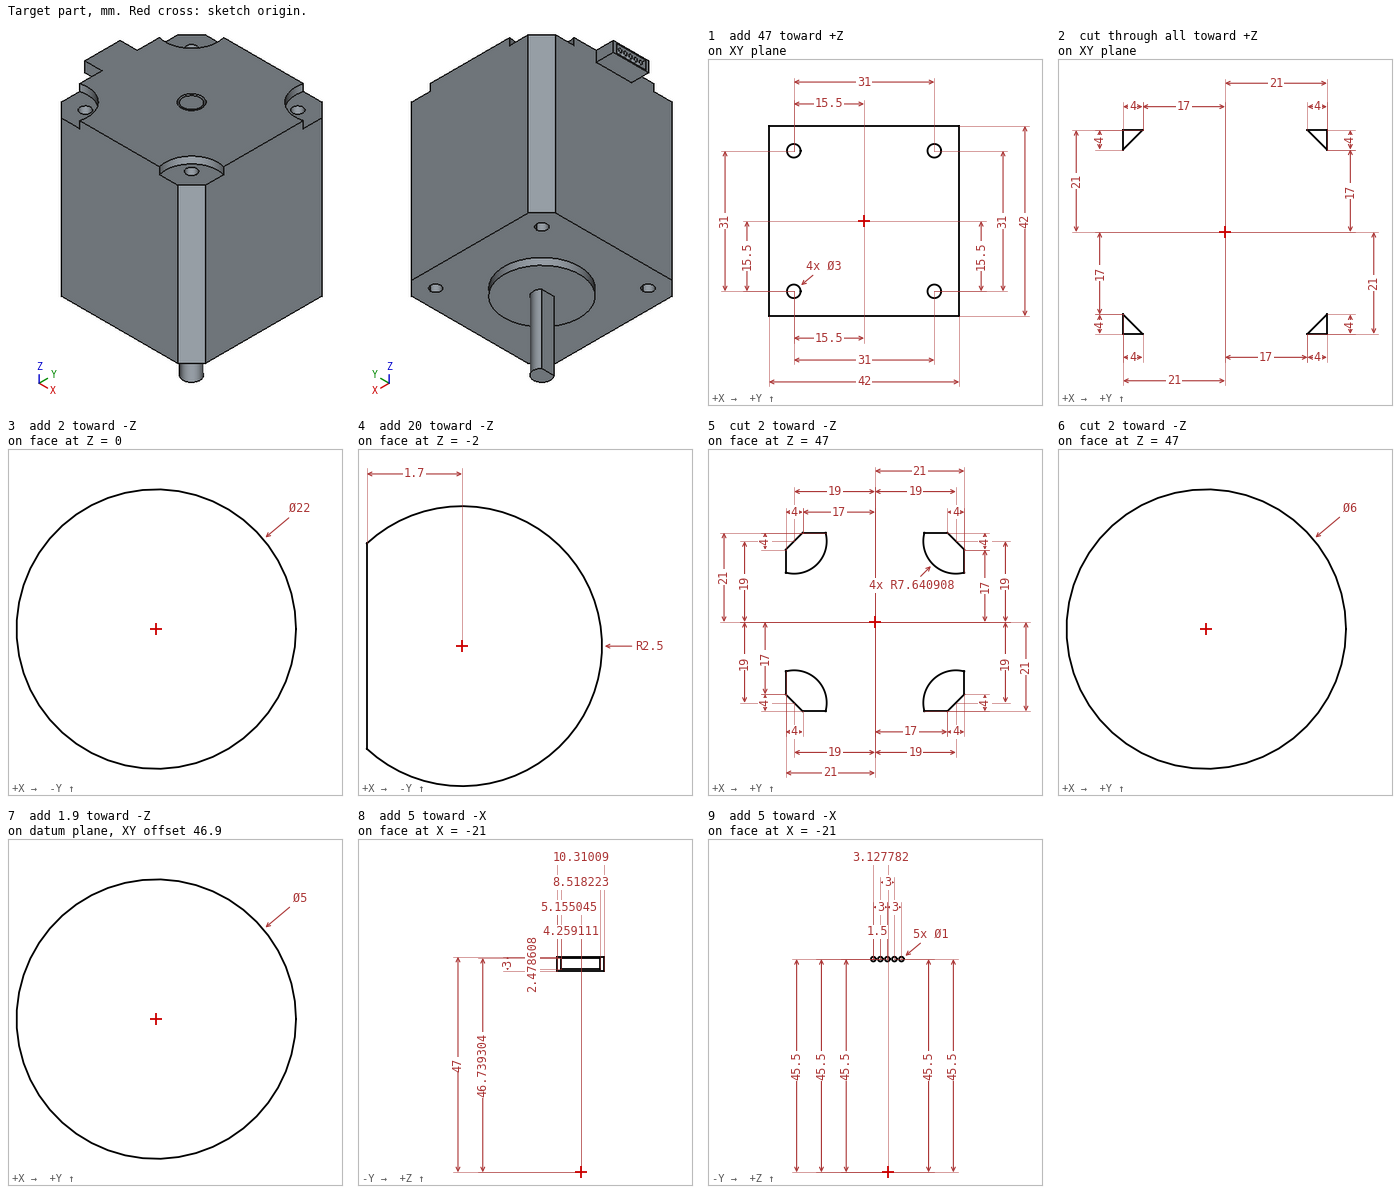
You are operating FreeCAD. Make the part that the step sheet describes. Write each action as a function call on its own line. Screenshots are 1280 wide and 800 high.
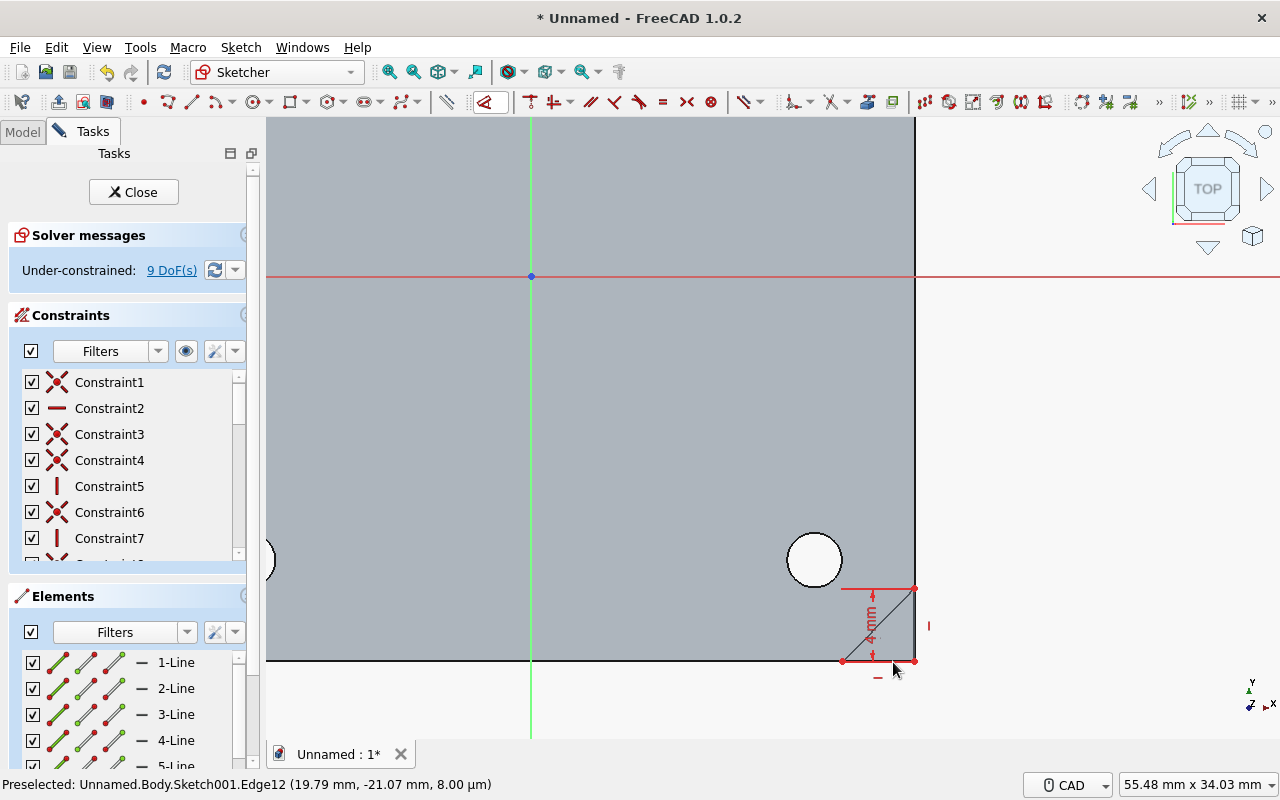
key(l)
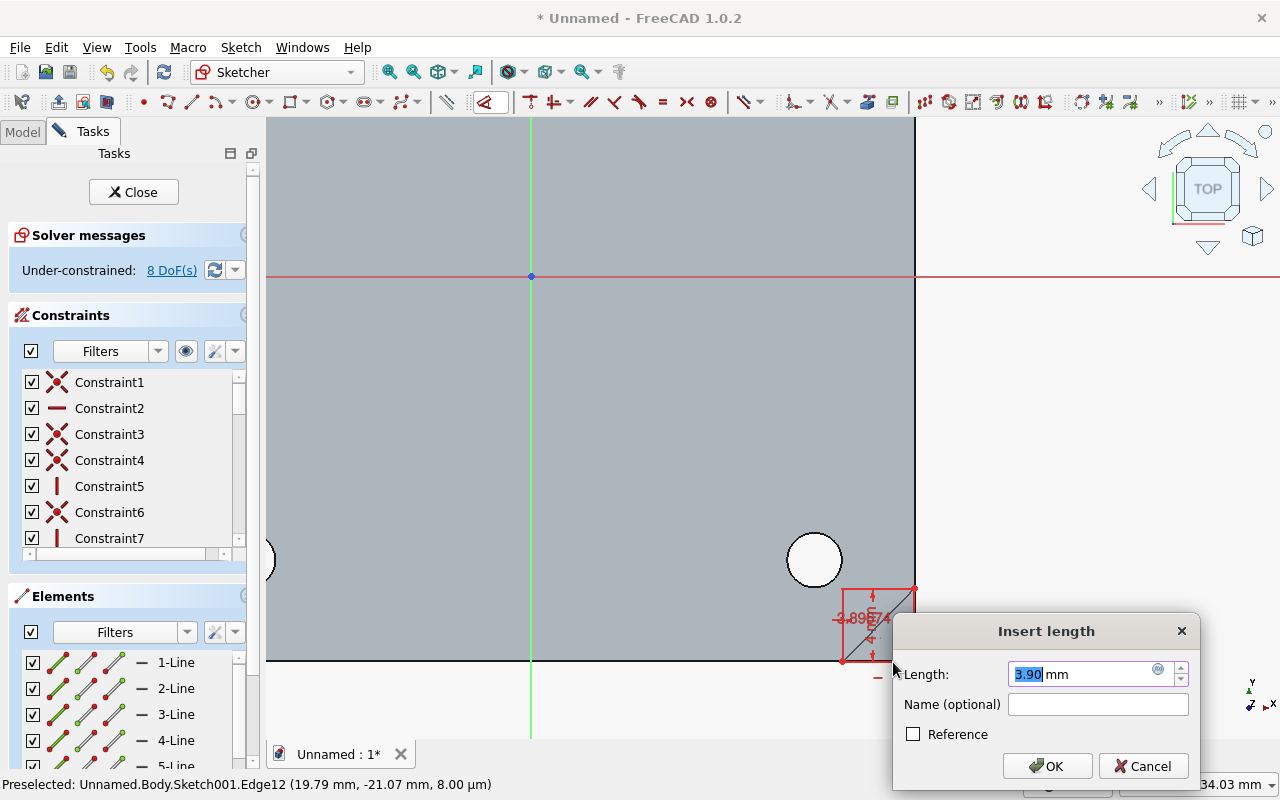
text(4)
key(Return)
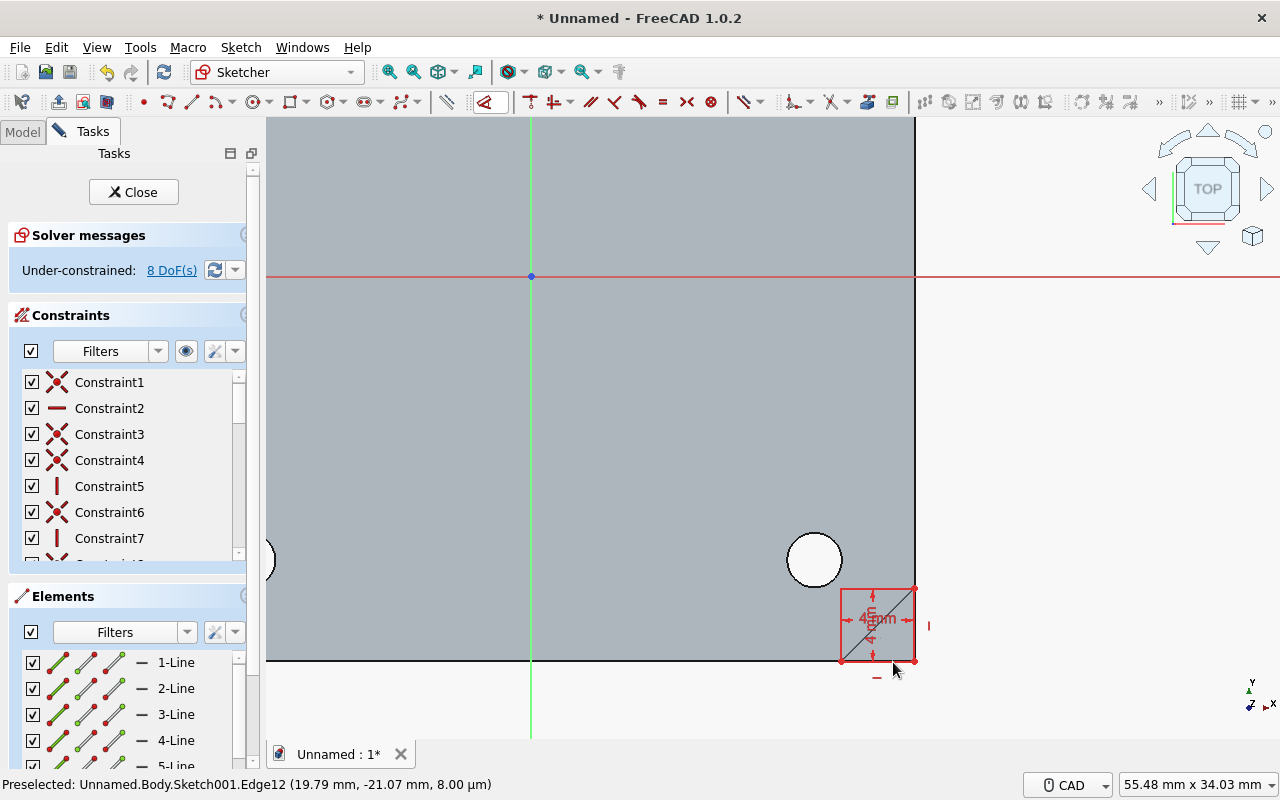
scroll(915, 612, down, 3)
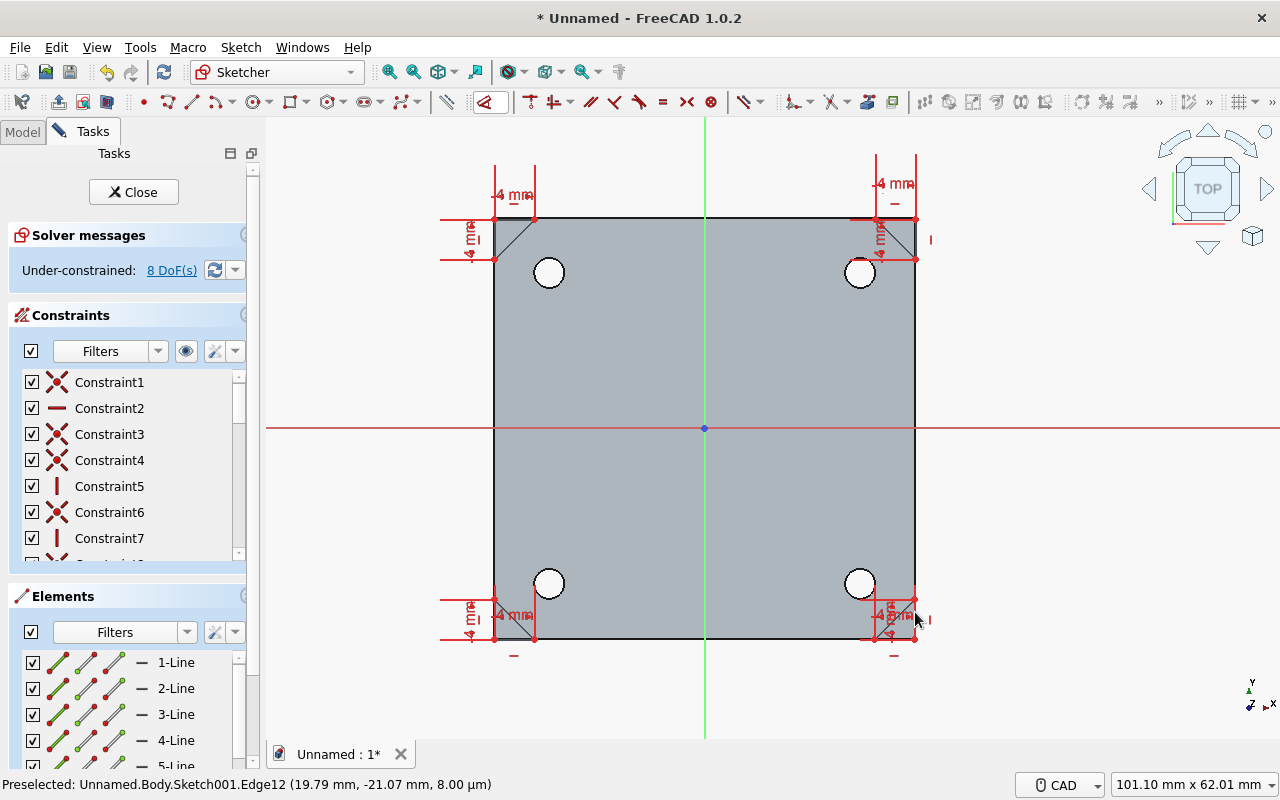
click(916, 260)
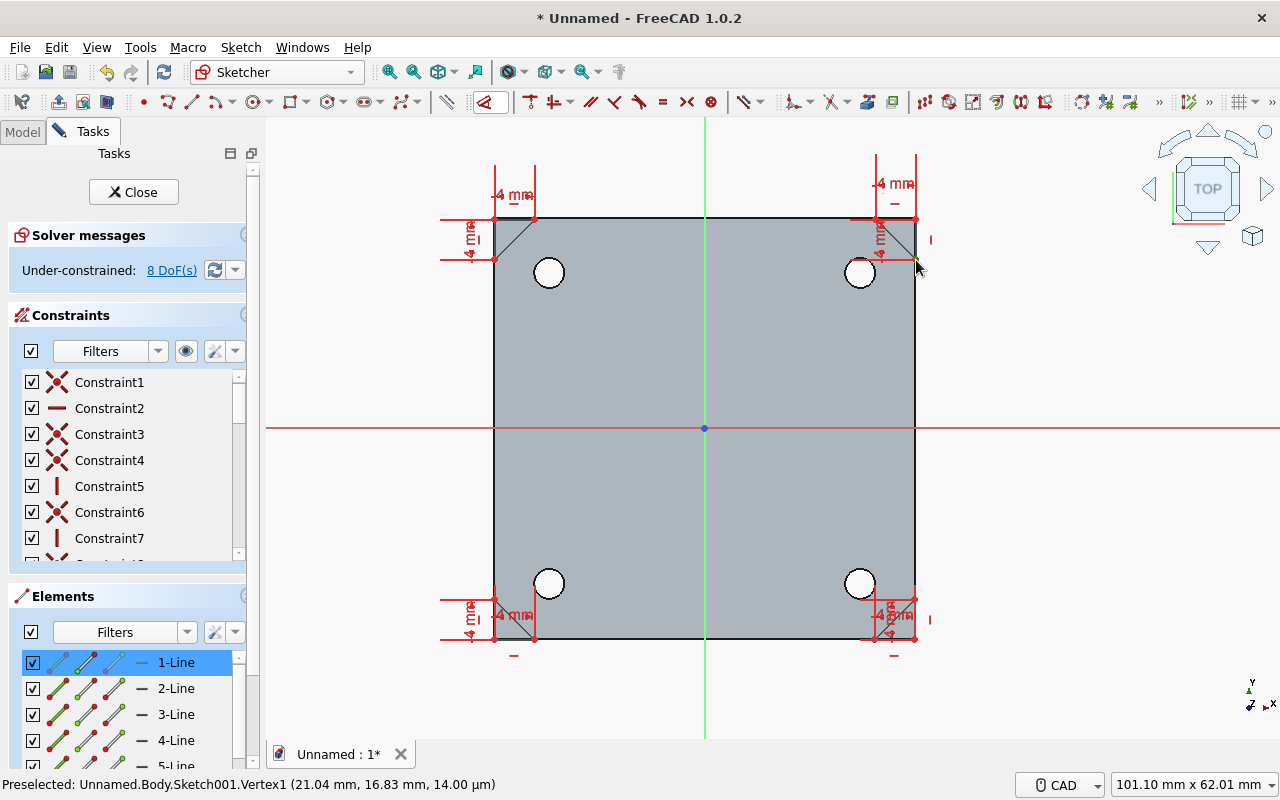
click(502, 102)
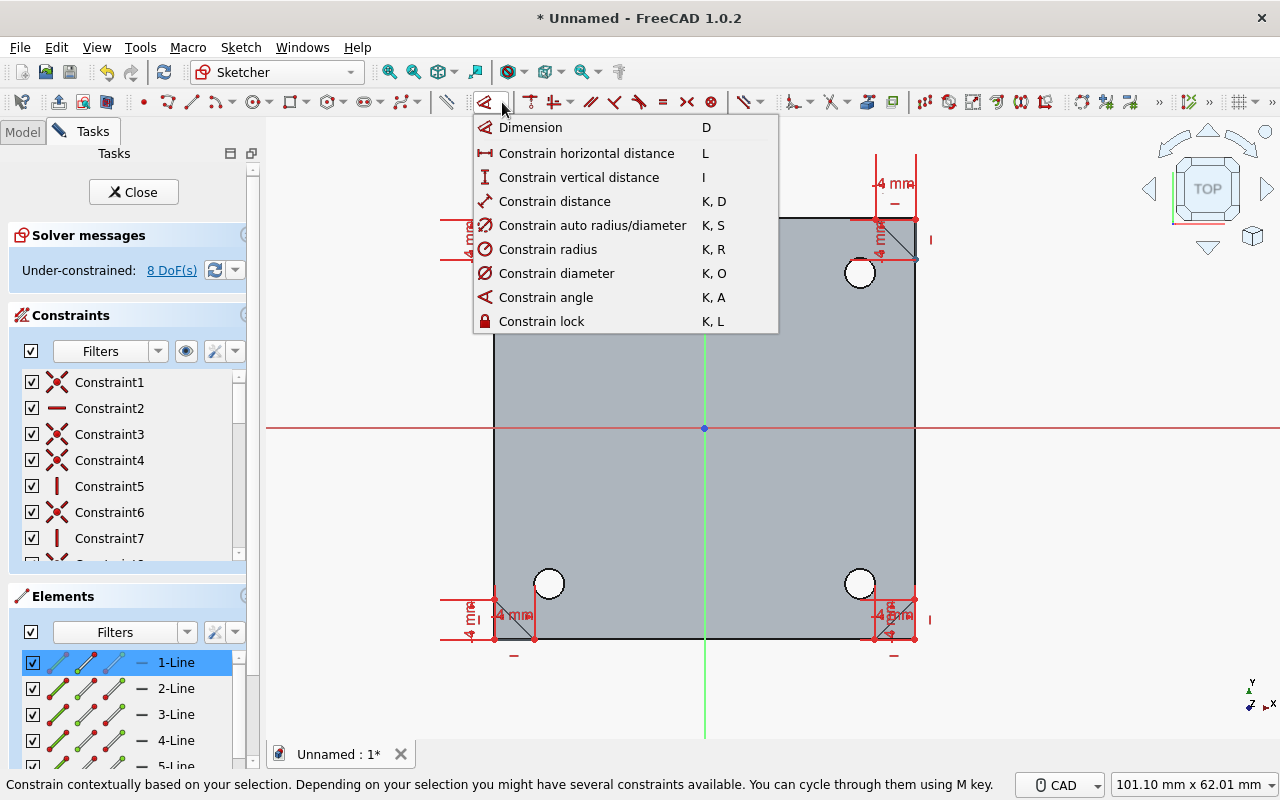
click(626, 153)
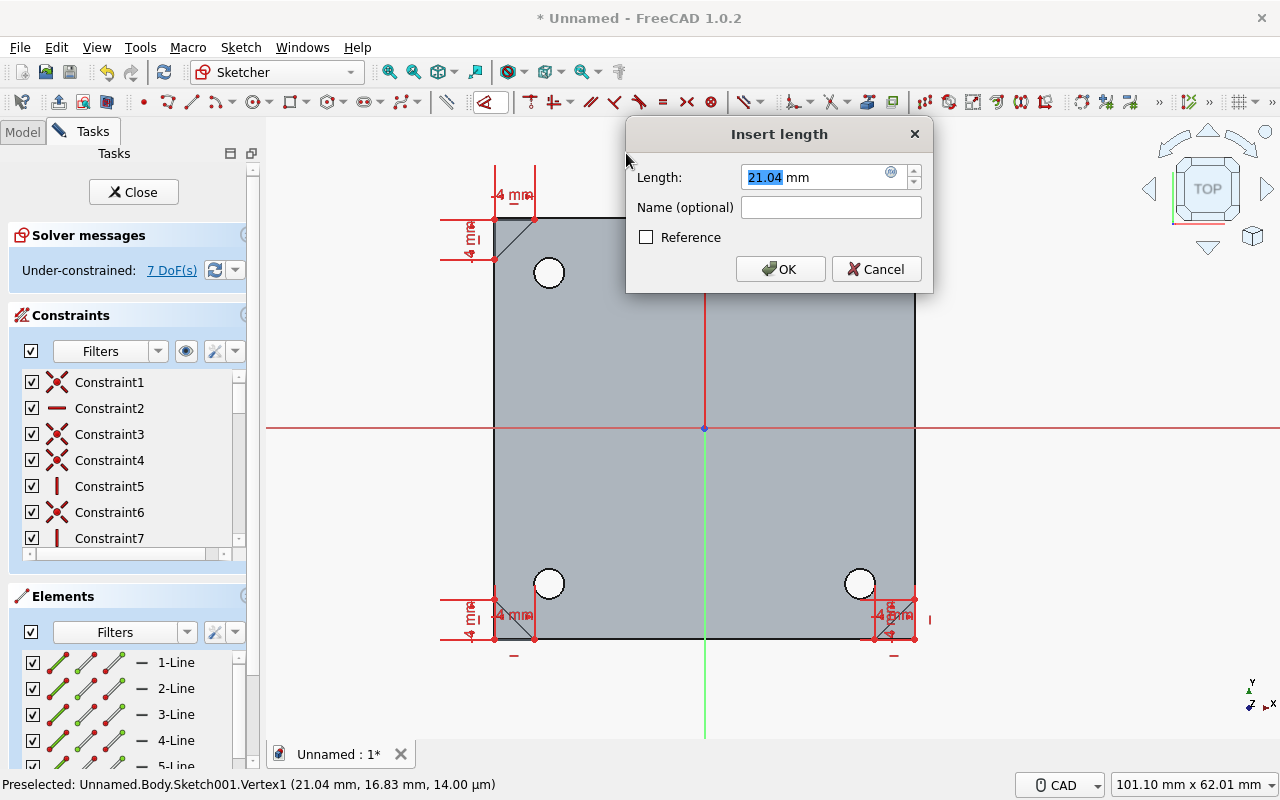
text(21)
key(Return)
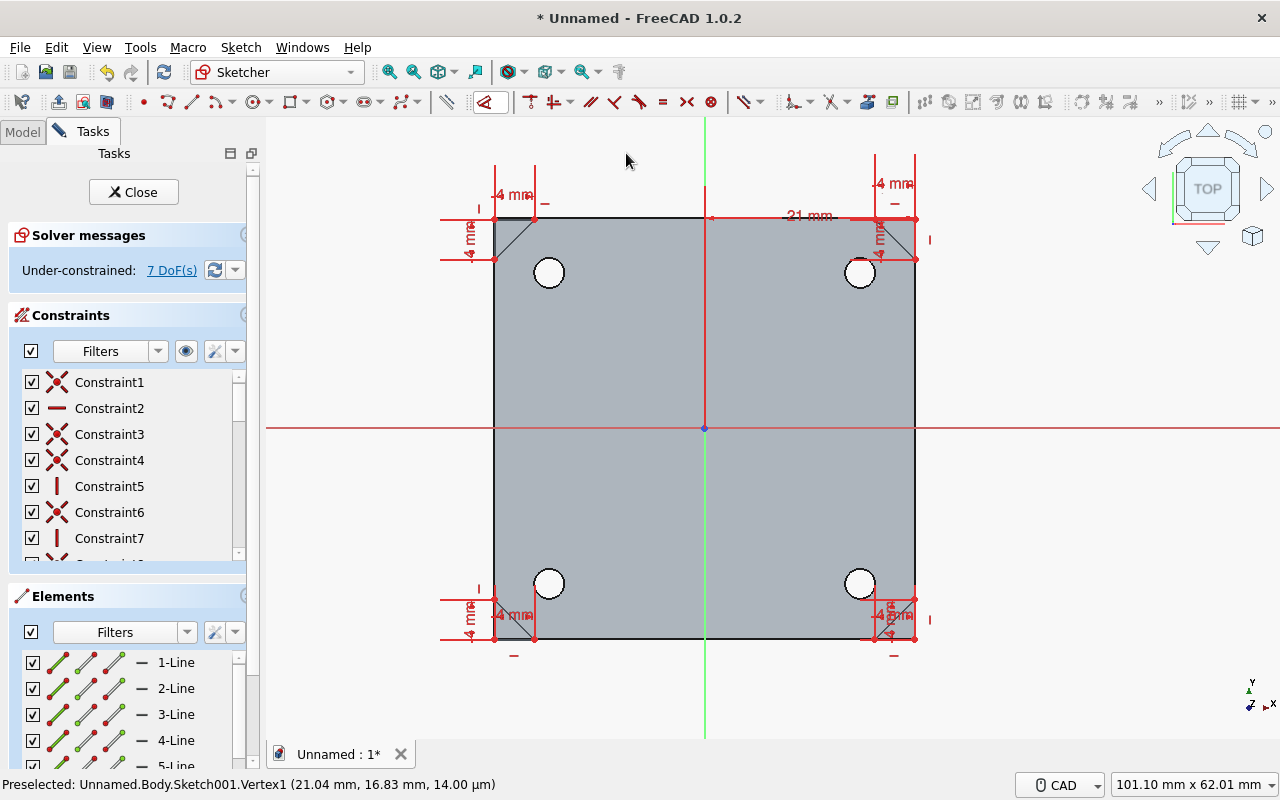
click(915, 260)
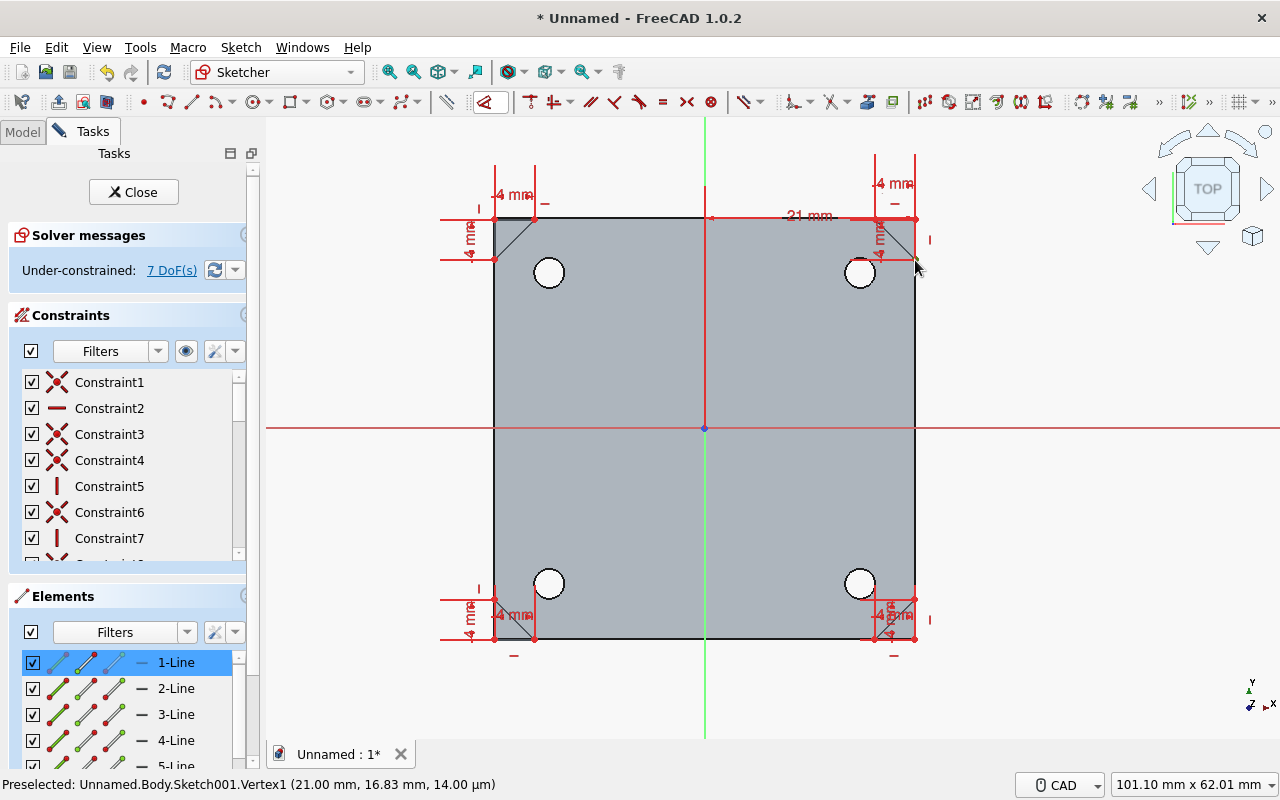
key(i)